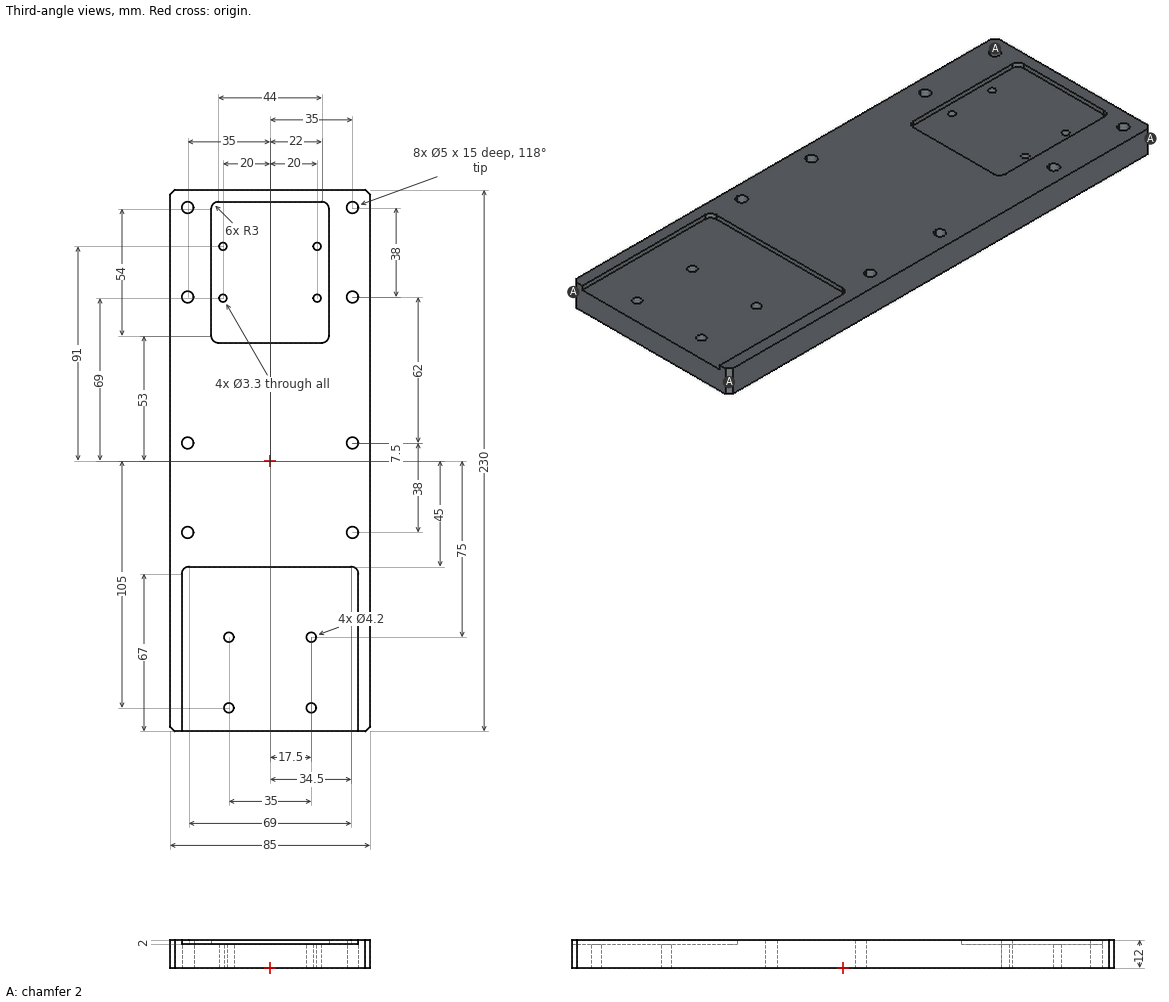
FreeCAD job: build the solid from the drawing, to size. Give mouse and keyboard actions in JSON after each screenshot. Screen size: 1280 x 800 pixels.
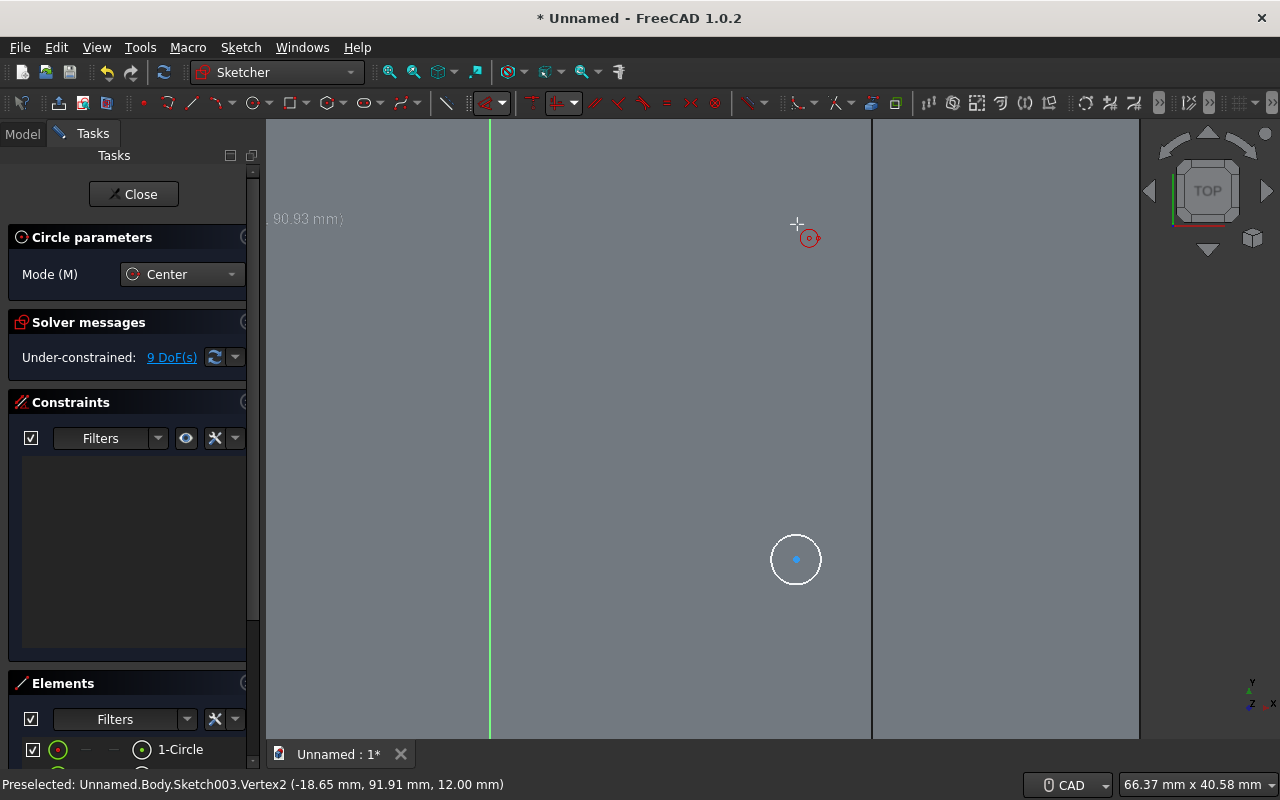
{"action": "left_click", "coordinate": [796, 223]}
{"action": "left_click", "coordinate": [814, 205]}
{"action": "key", "text": "Escape"}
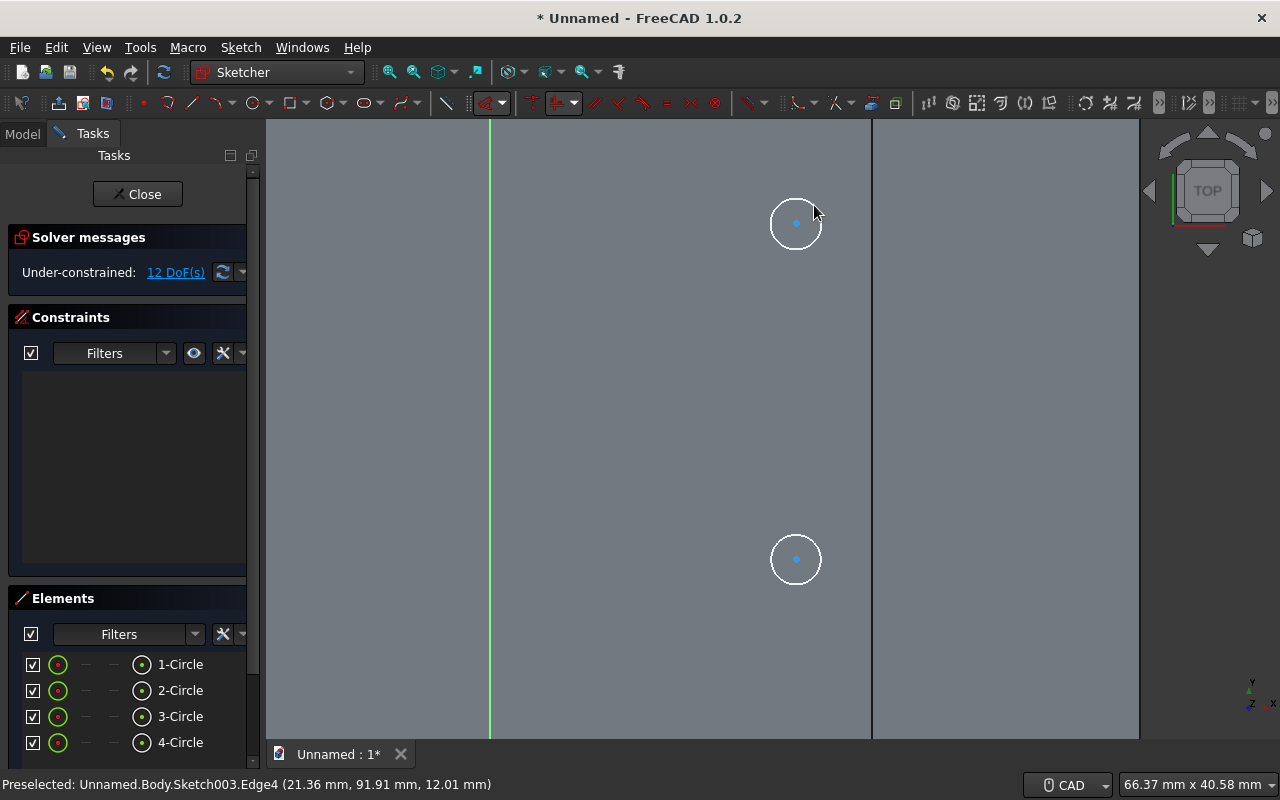
{"action": "scroll", "coordinate": [797, 224], "scroll_direction": "down", "scroll_amount": 6}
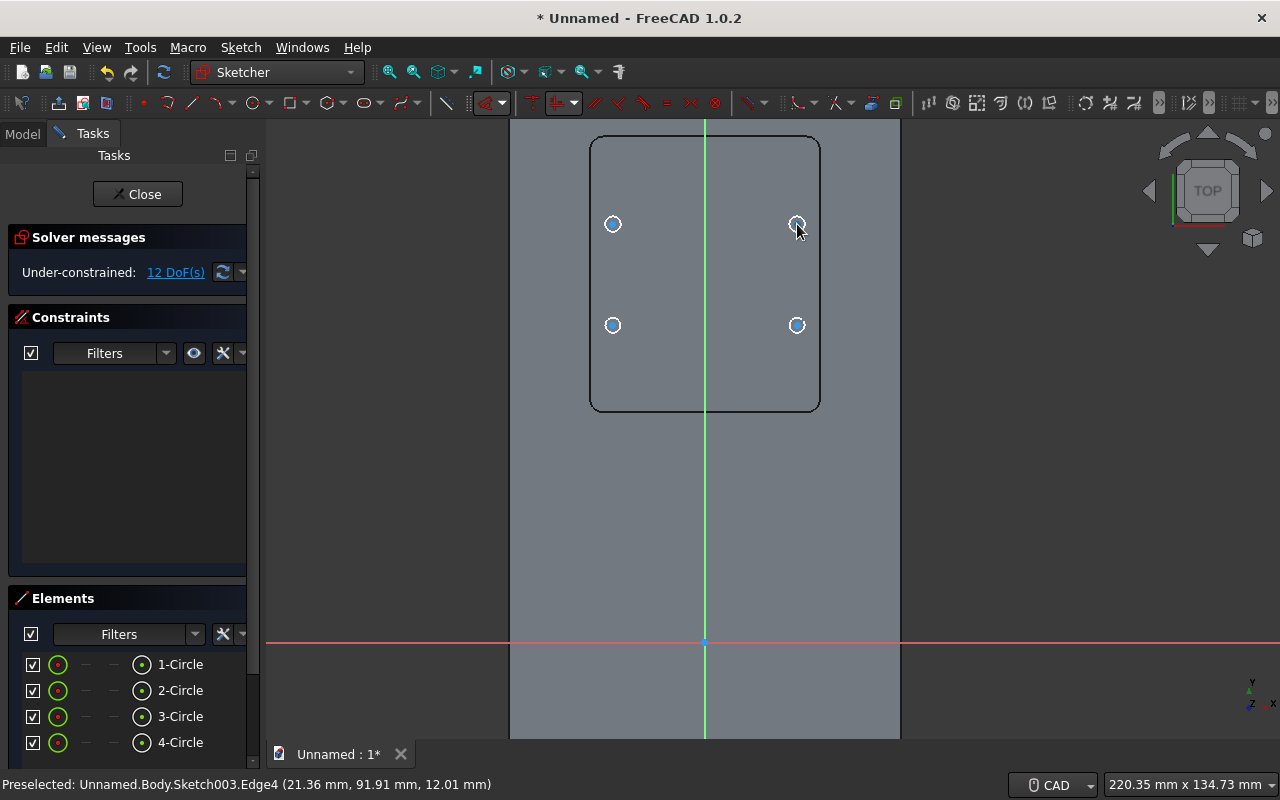
{"action": "scroll", "coordinate": [618, 320], "scroll_direction": "up", "scroll_amount": 4}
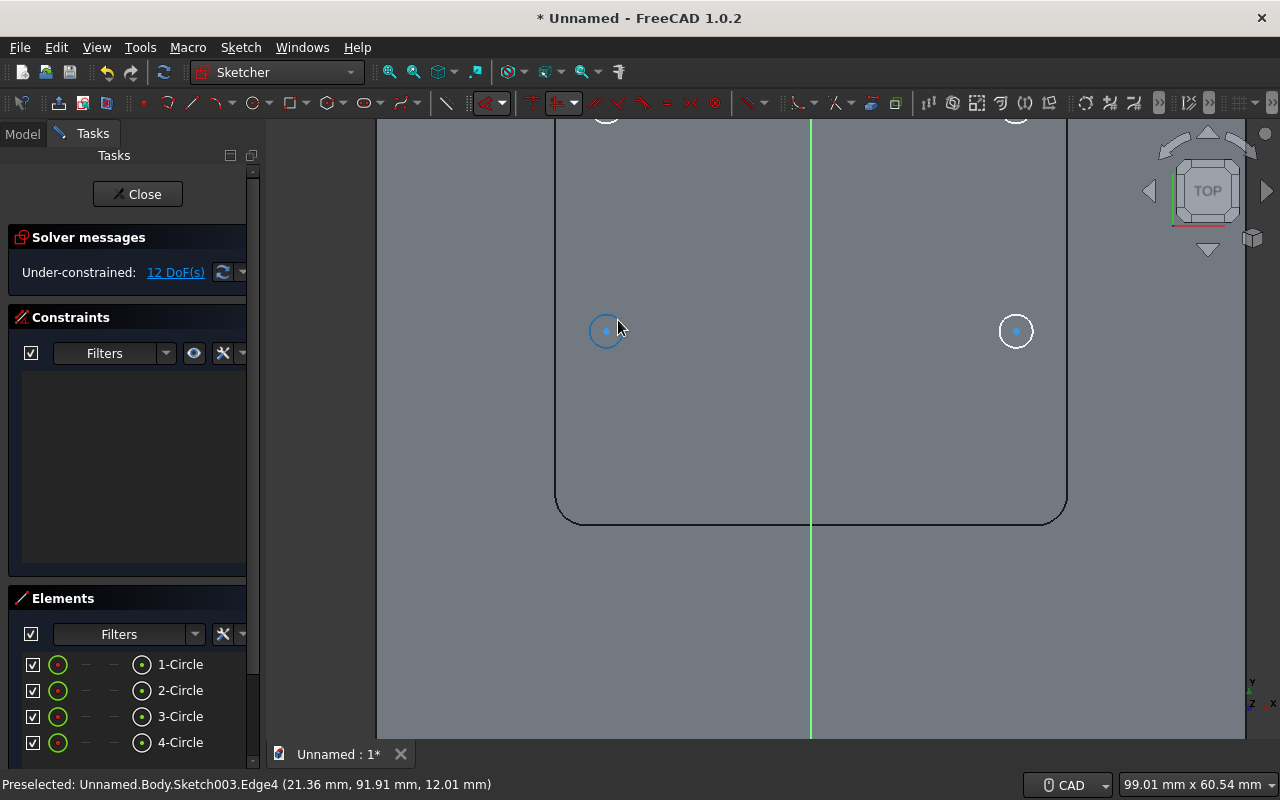
{"action": "left_click", "coordinate": [618, 319]}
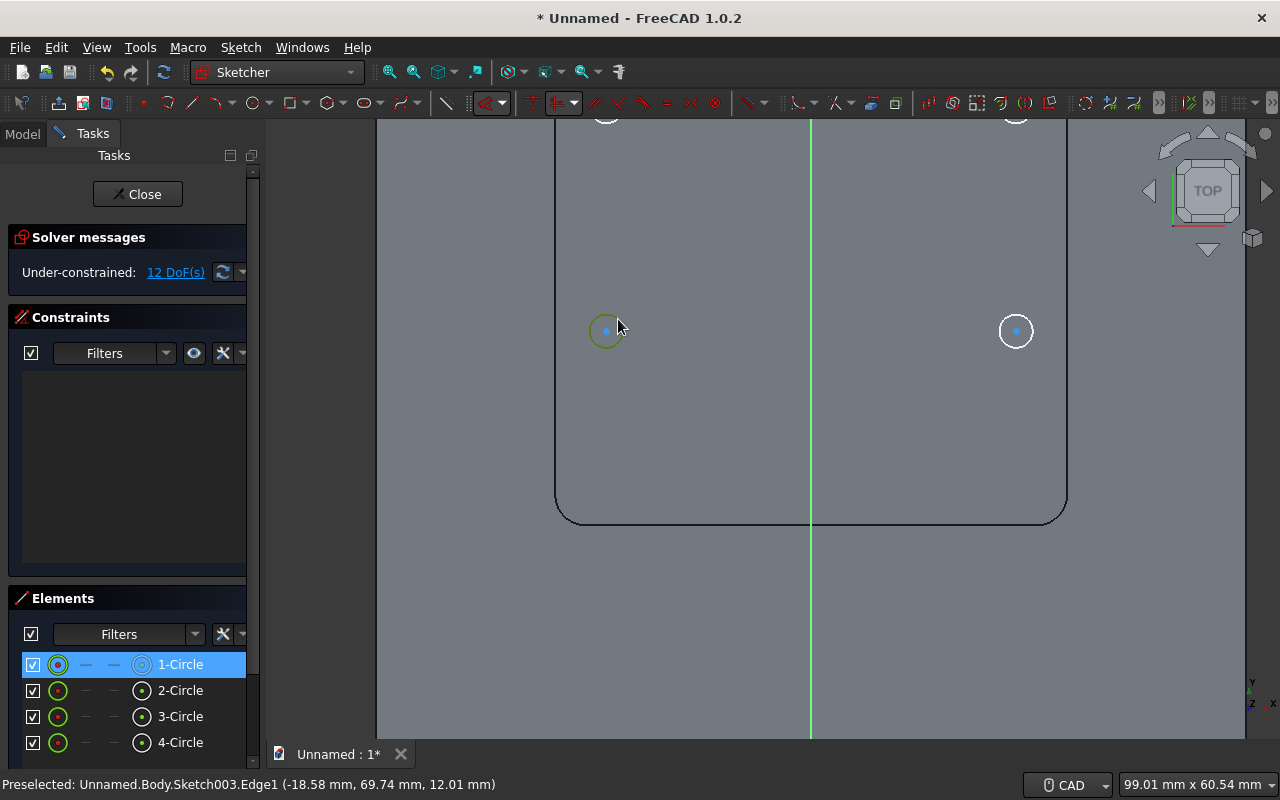
{"action": "left_click", "coordinate": [1028, 319]}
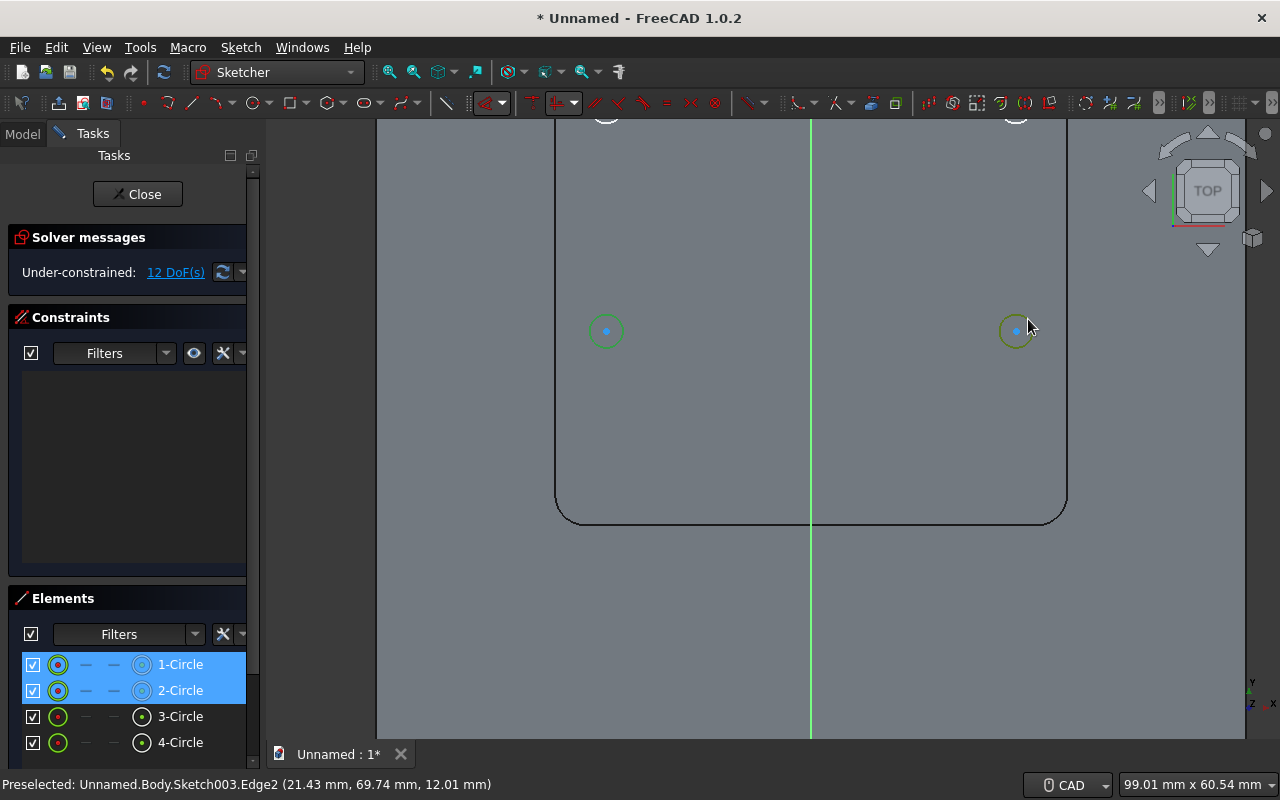
{"action": "scroll", "coordinate": [617, 320], "scroll_direction": "down", "scroll_amount": 4}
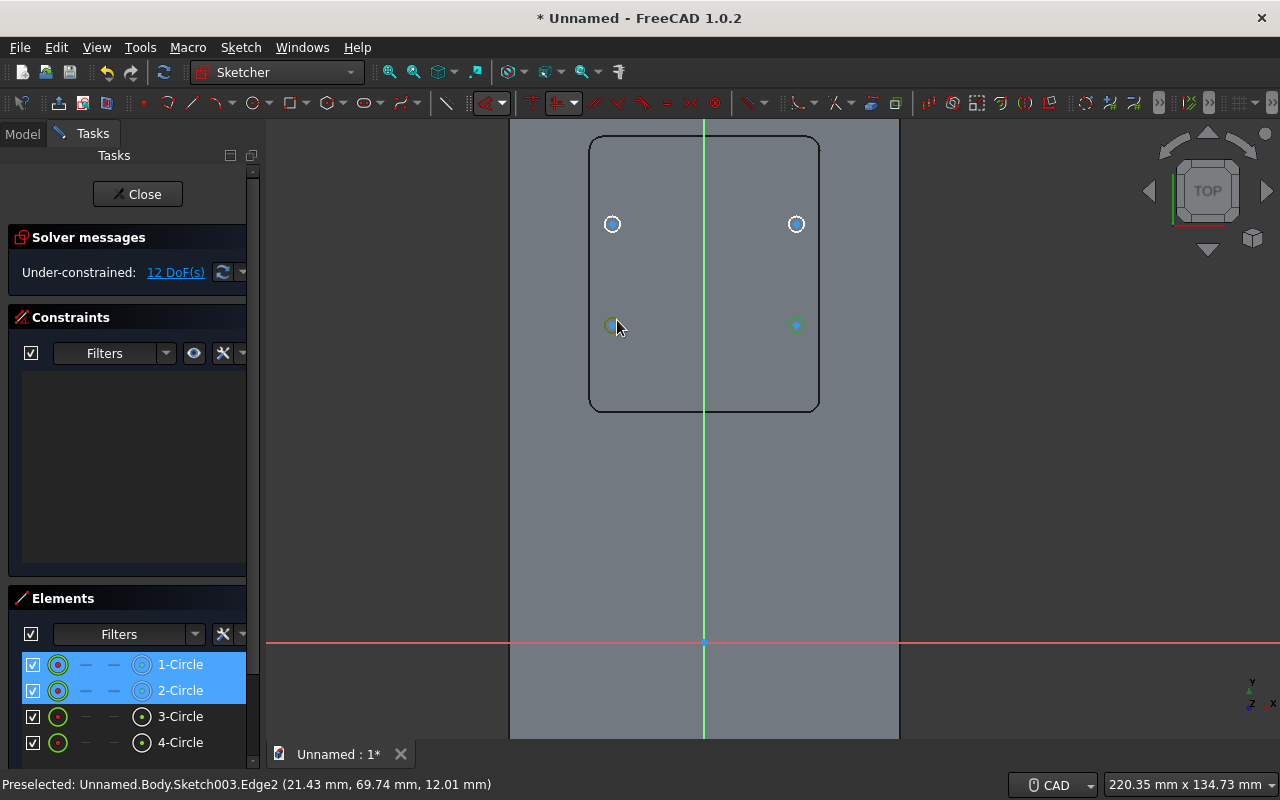
{"action": "scroll", "coordinate": [618, 219], "scroll_direction": "up", "scroll_amount": 3}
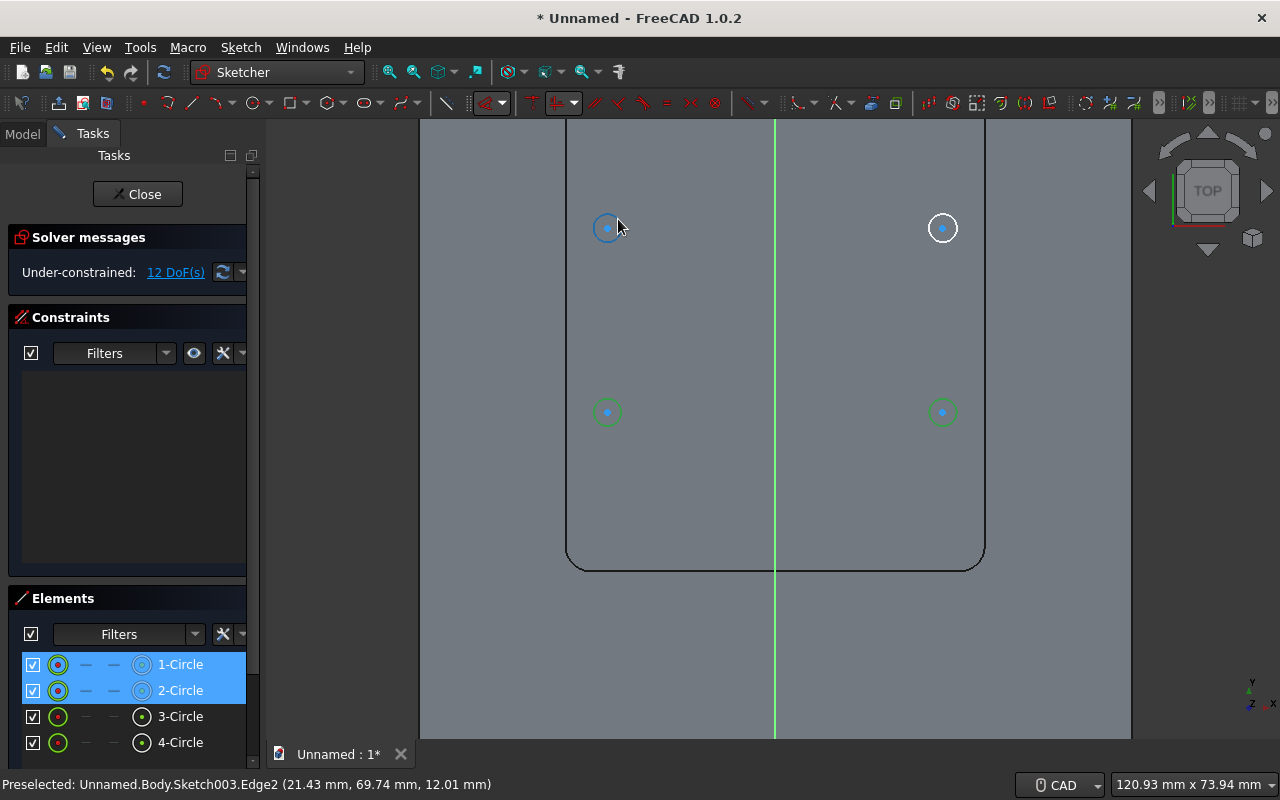
{"action": "left_click", "coordinate": [617, 218]}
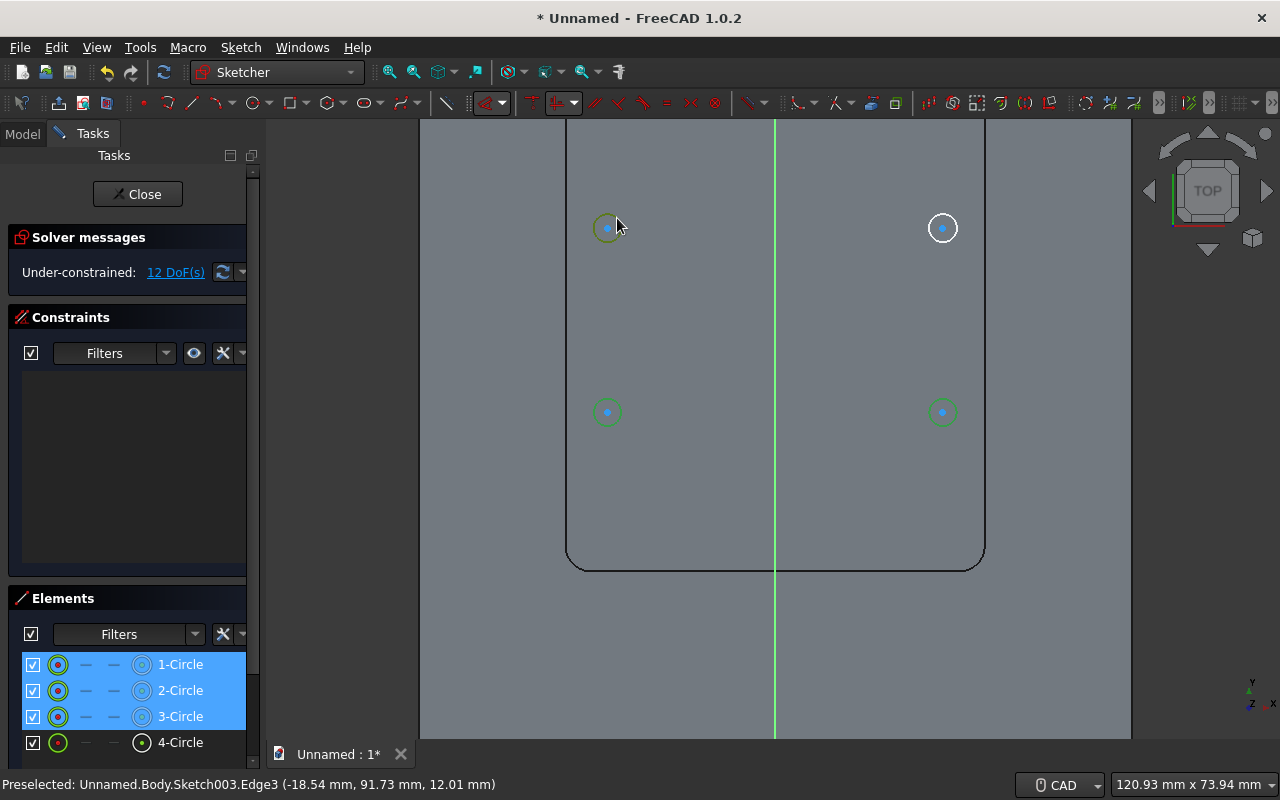
{"action": "left_click", "coordinate": [953, 218]}